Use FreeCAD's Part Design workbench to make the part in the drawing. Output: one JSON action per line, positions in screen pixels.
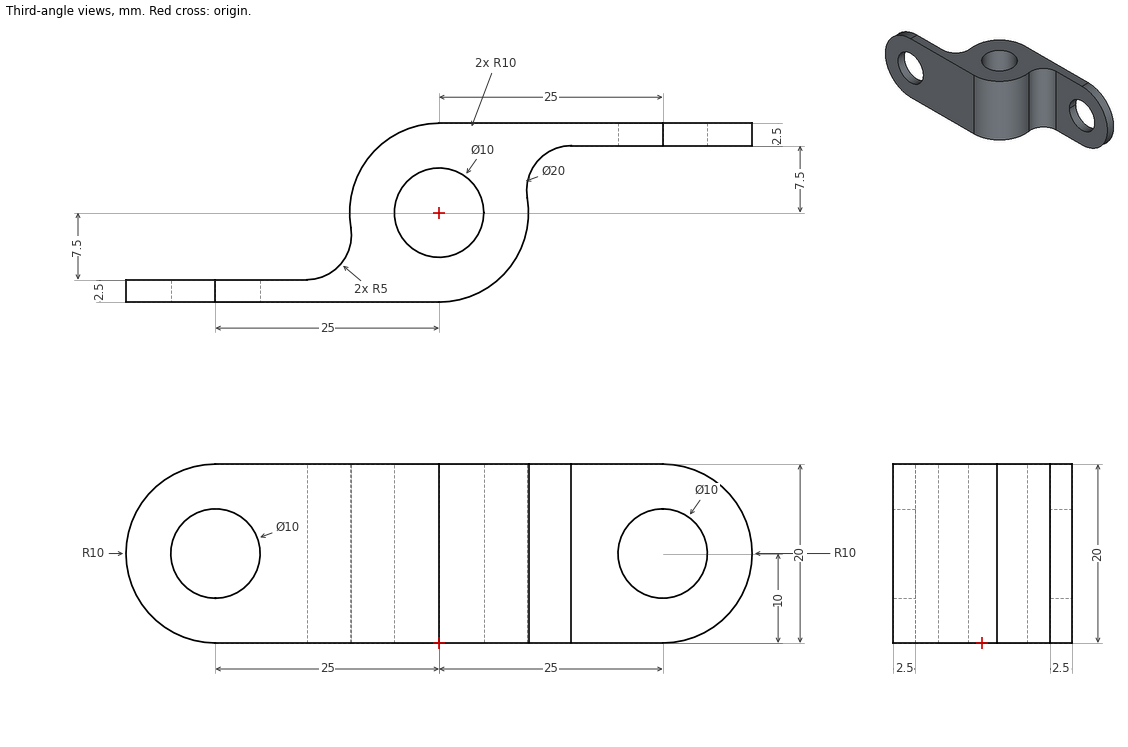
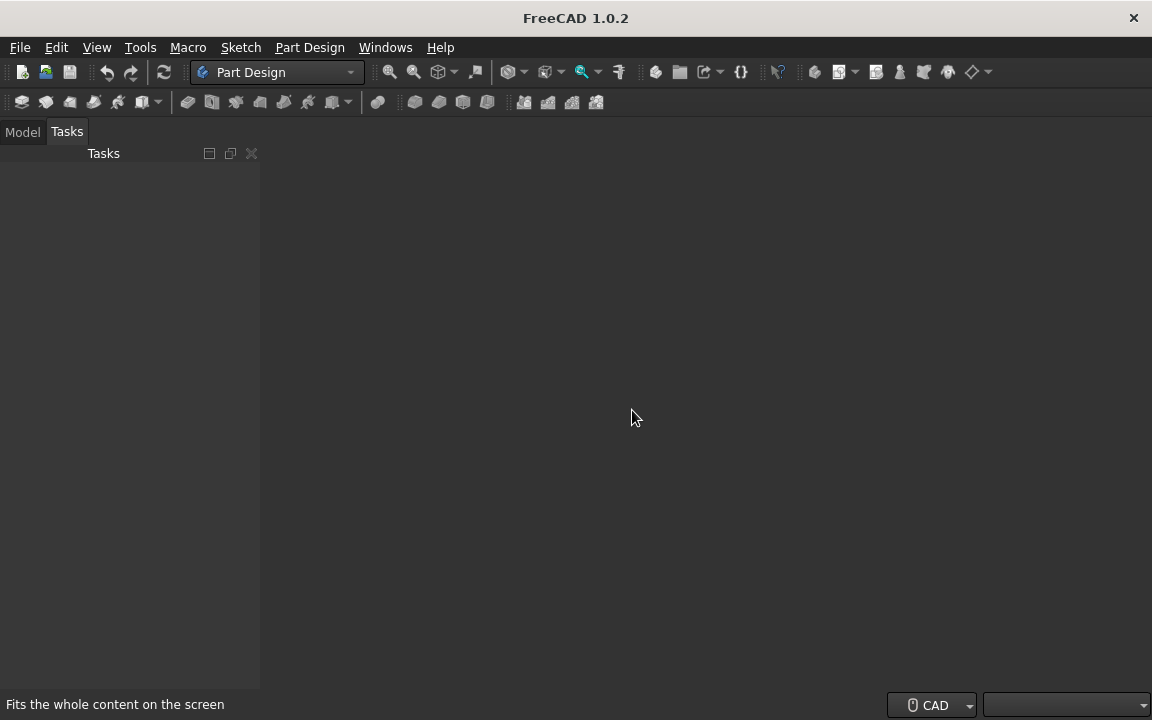
{"action": "key", "text": "ctrl+n"}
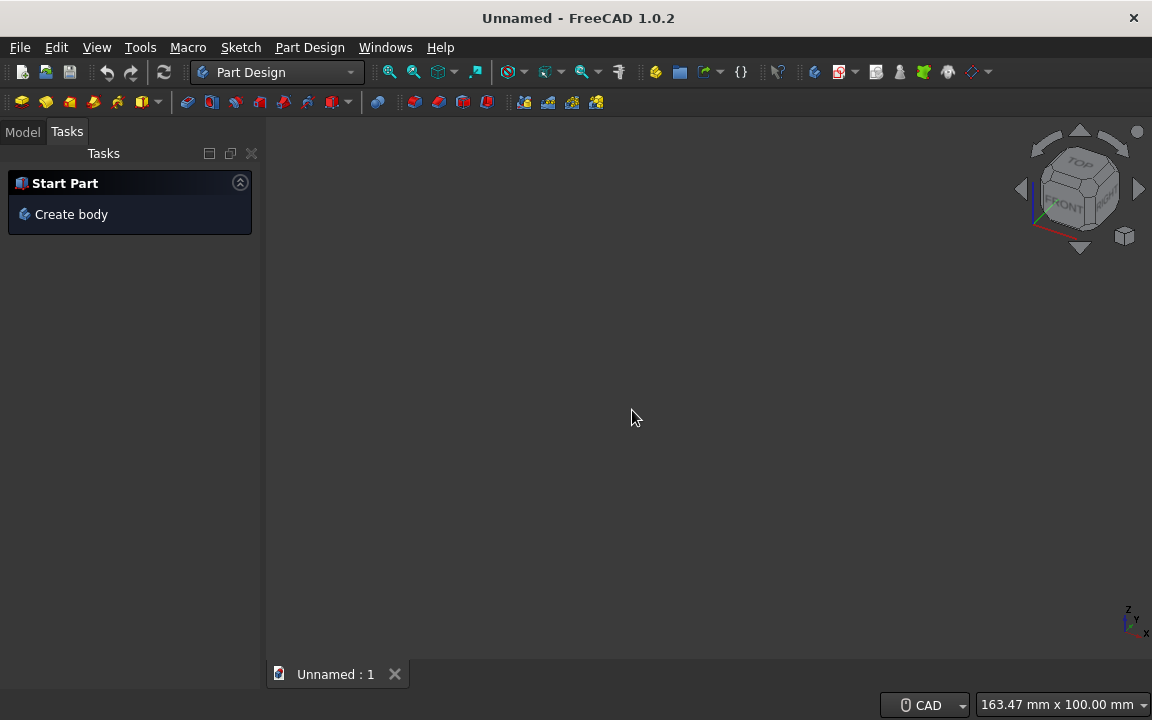
{"action": "left_click", "coordinate": [840, 72]}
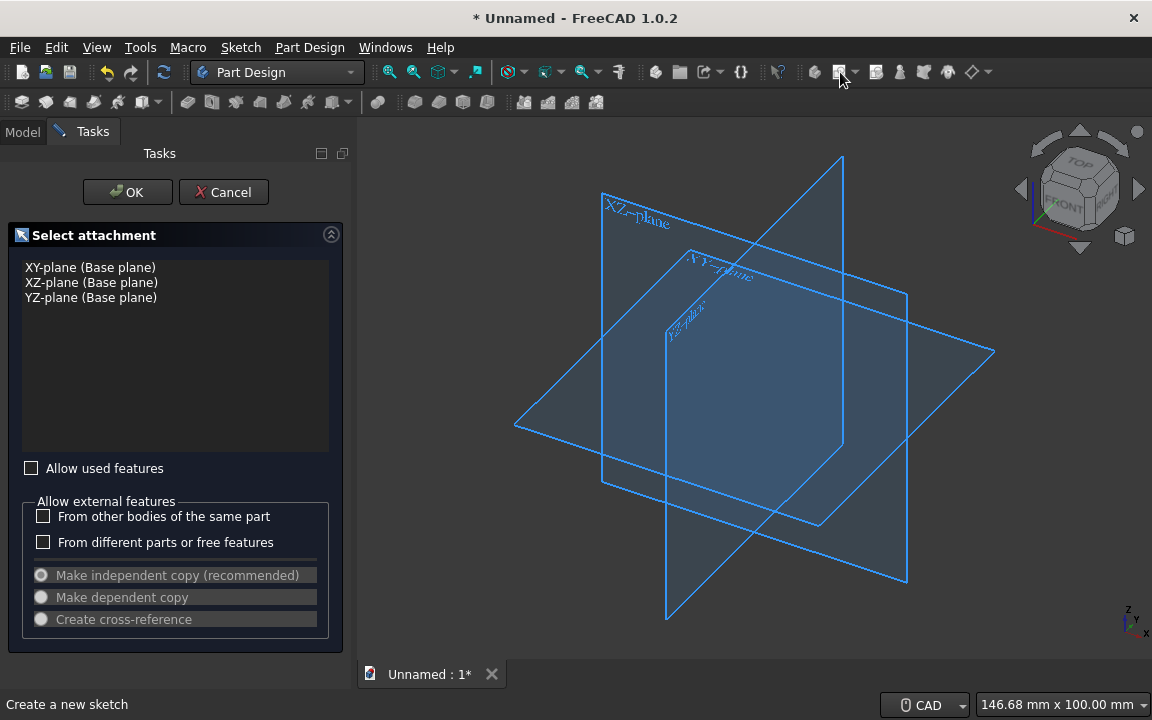
{"action": "left_click", "coordinate": [82, 268]}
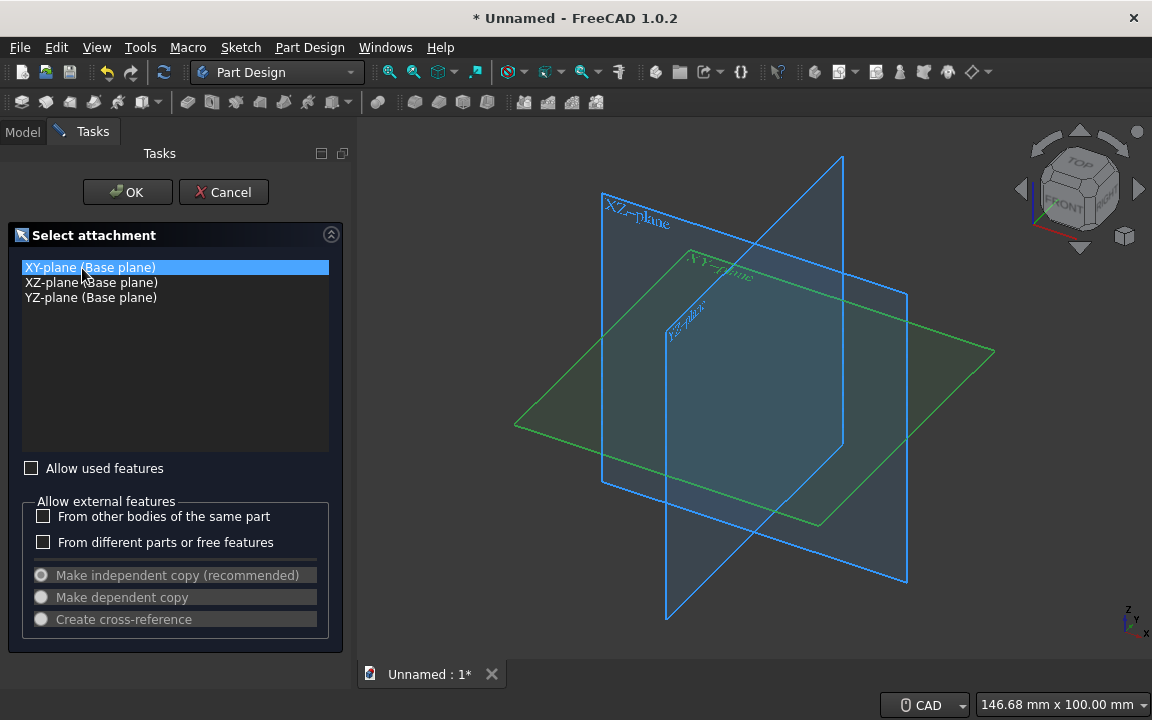
{"action": "left_click", "coordinate": [128, 192]}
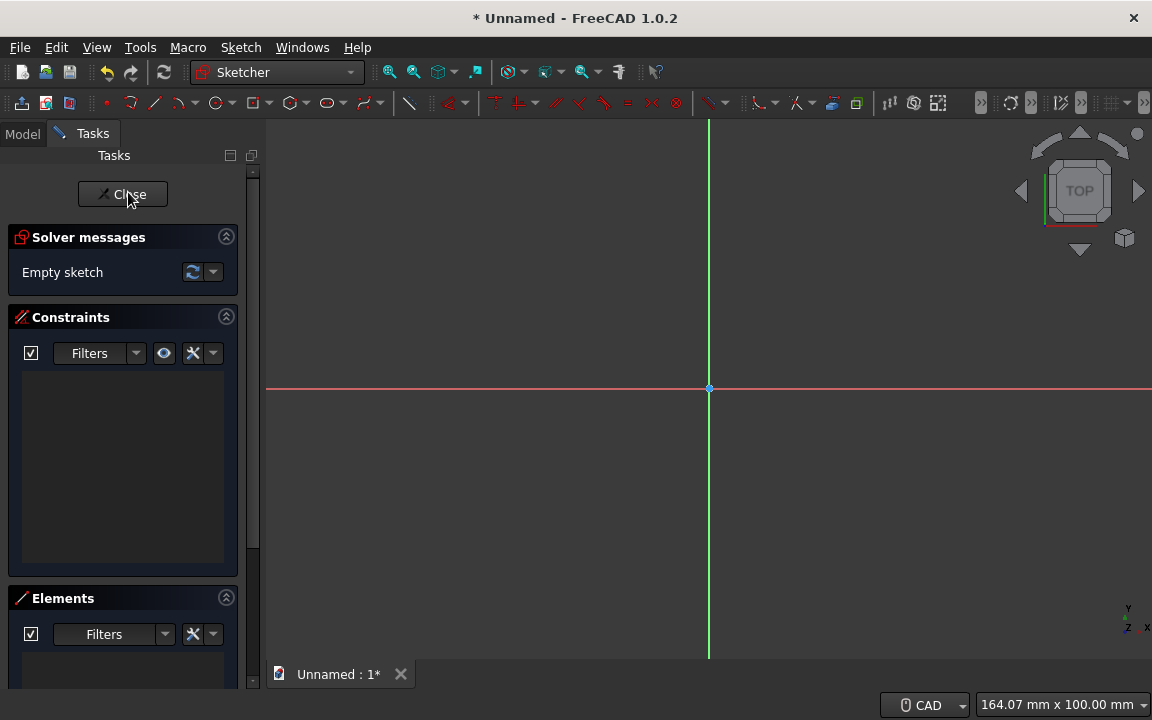
{"action": "scroll", "coordinate": [739, 389], "scroll_direction": "up", "scroll_amount": 6}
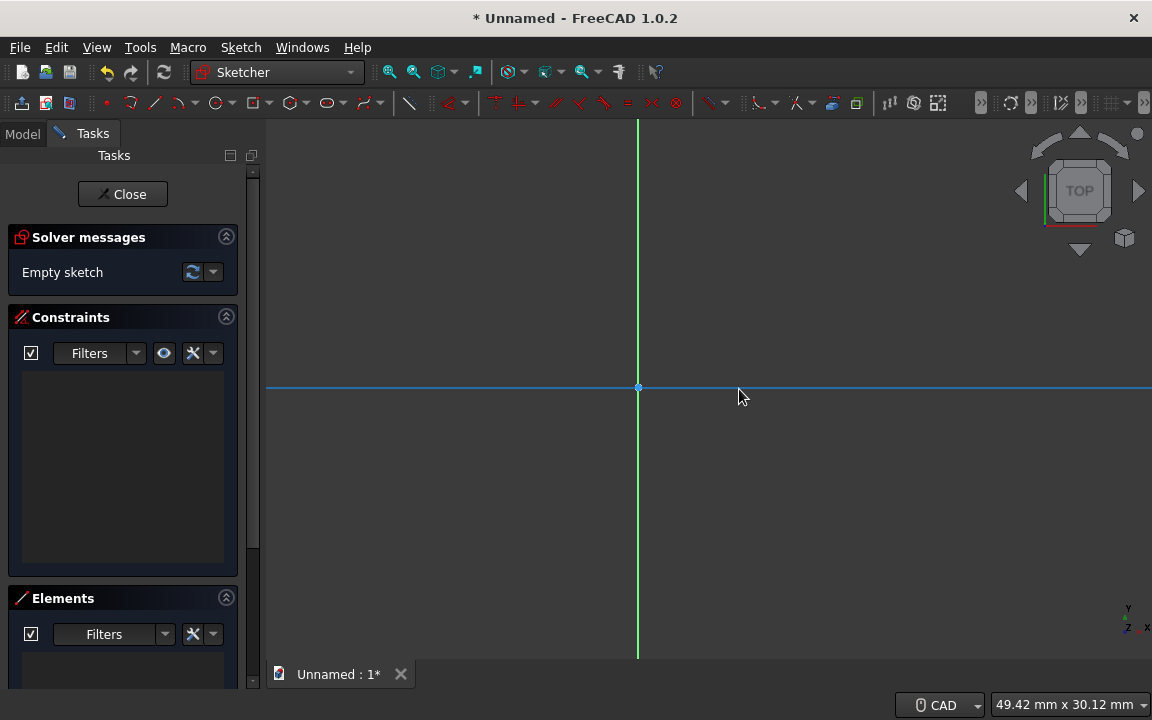
{"action": "key", "text": "g c"}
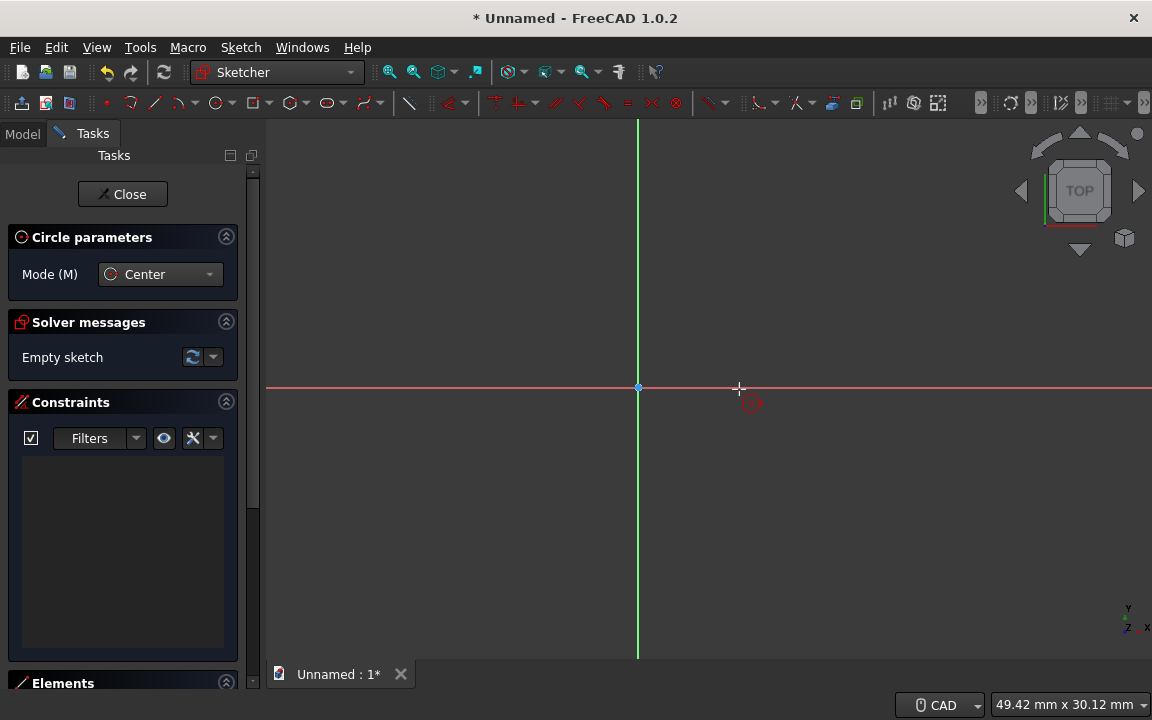
{"action": "left_click", "coordinate": [638, 388]}
{"action": "left_click", "coordinate": [765, 261]}
{"action": "key", "text": "Escape"}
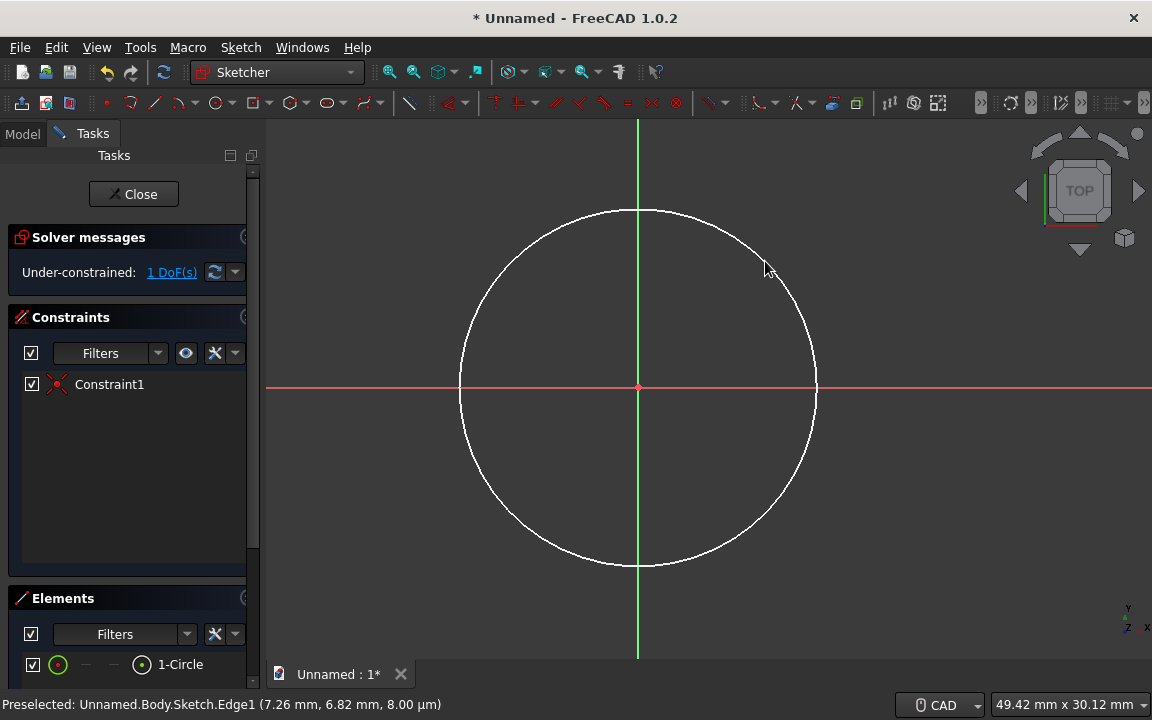
{"action": "key", "text": "d"}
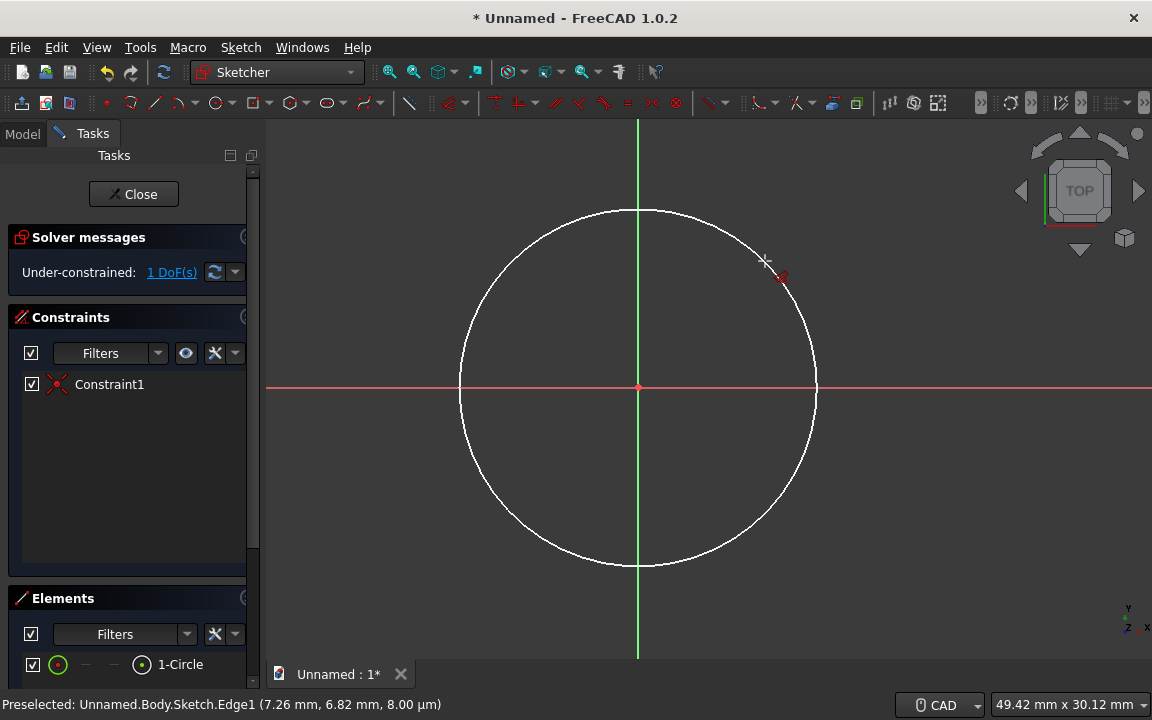
{"action": "left_click", "coordinate": [764, 261]}
{"action": "left_click", "coordinate": [787, 238]}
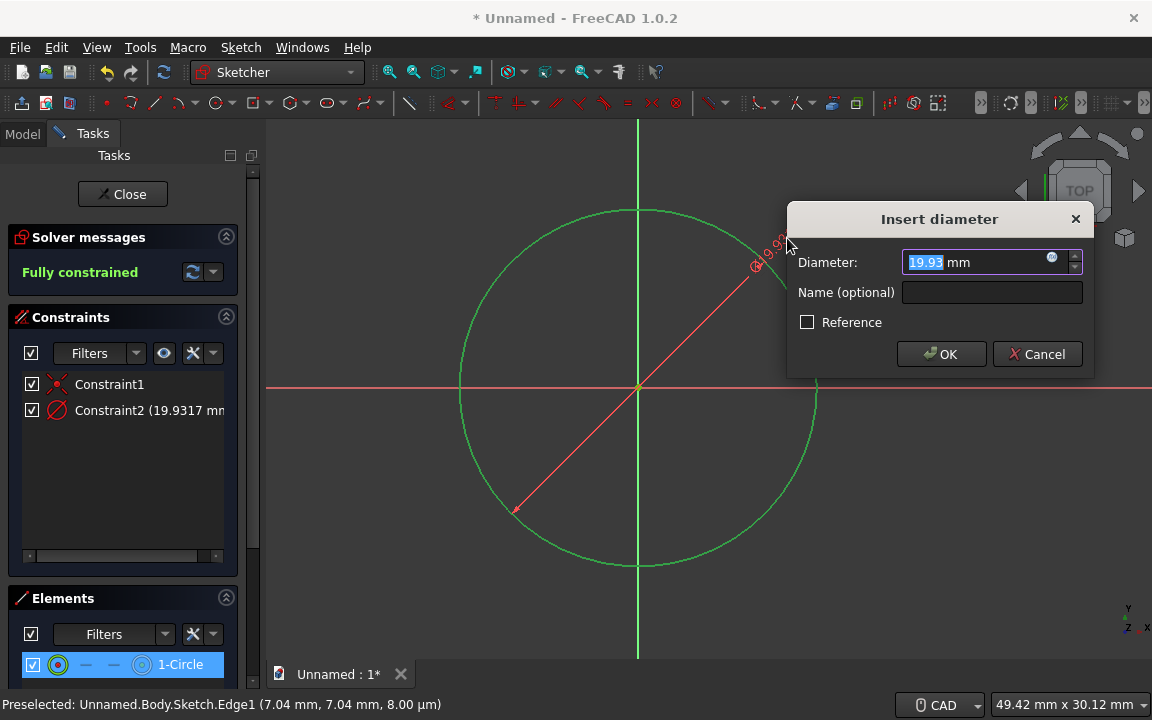
{"action": "type", "text": "20"}
{"action": "key", "text": "Return"}
{"action": "key", "text": "Escape"}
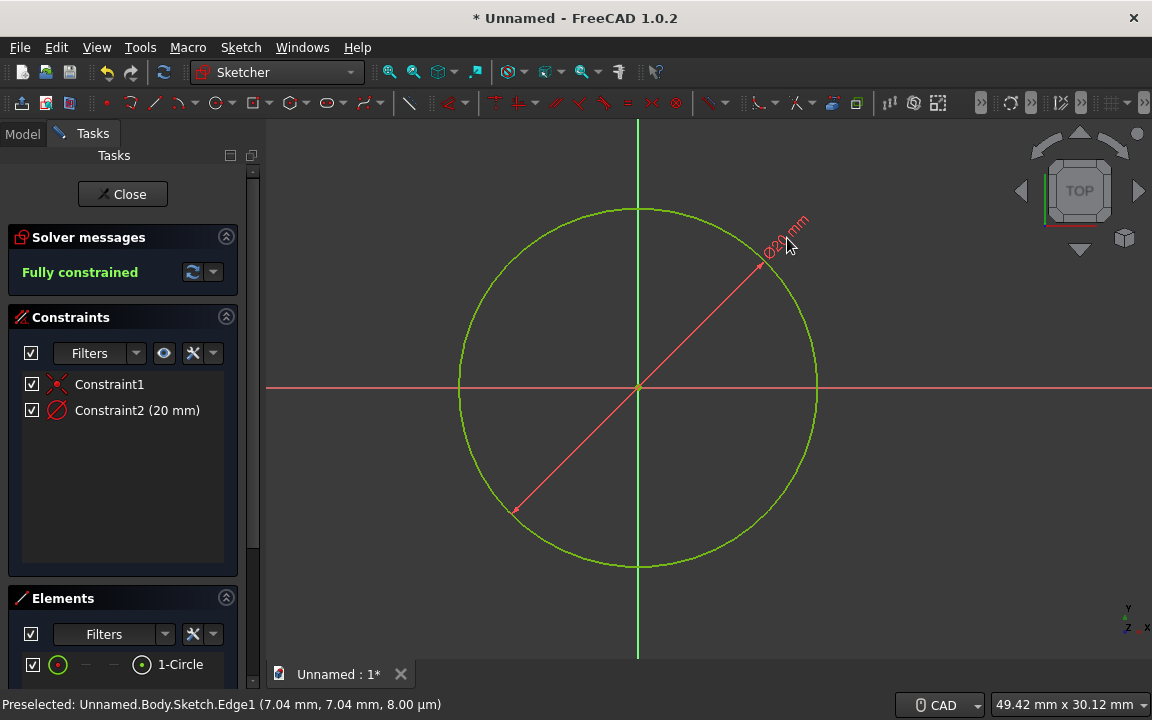
{"action": "left_click", "coordinate": [123, 194]}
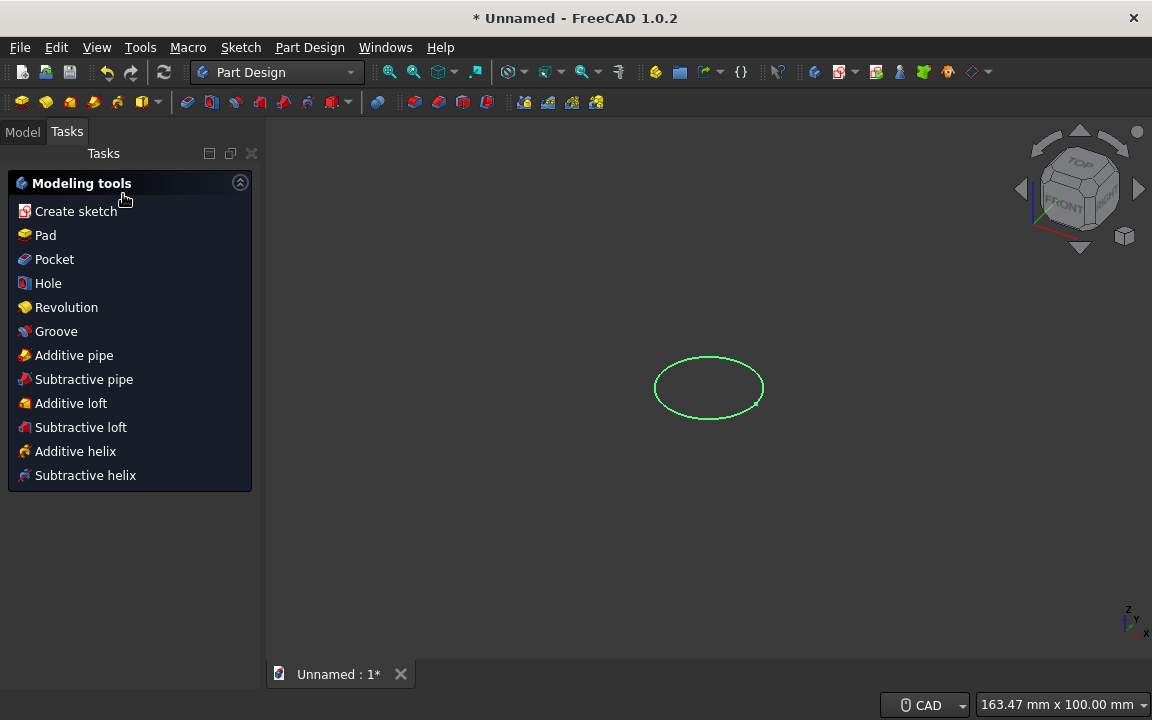
{"action": "left_click", "coordinate": [22, 102]}